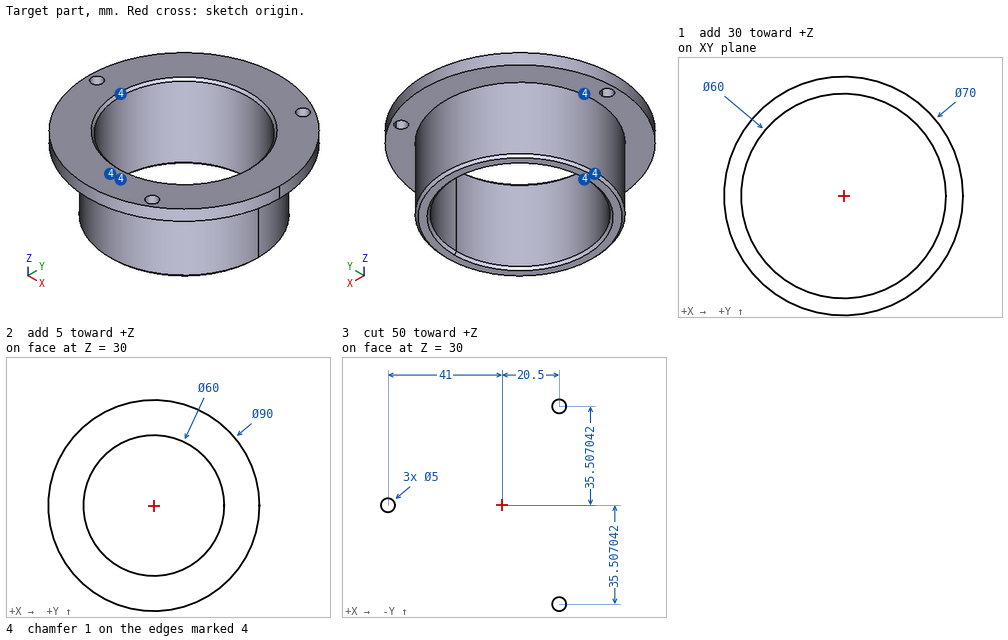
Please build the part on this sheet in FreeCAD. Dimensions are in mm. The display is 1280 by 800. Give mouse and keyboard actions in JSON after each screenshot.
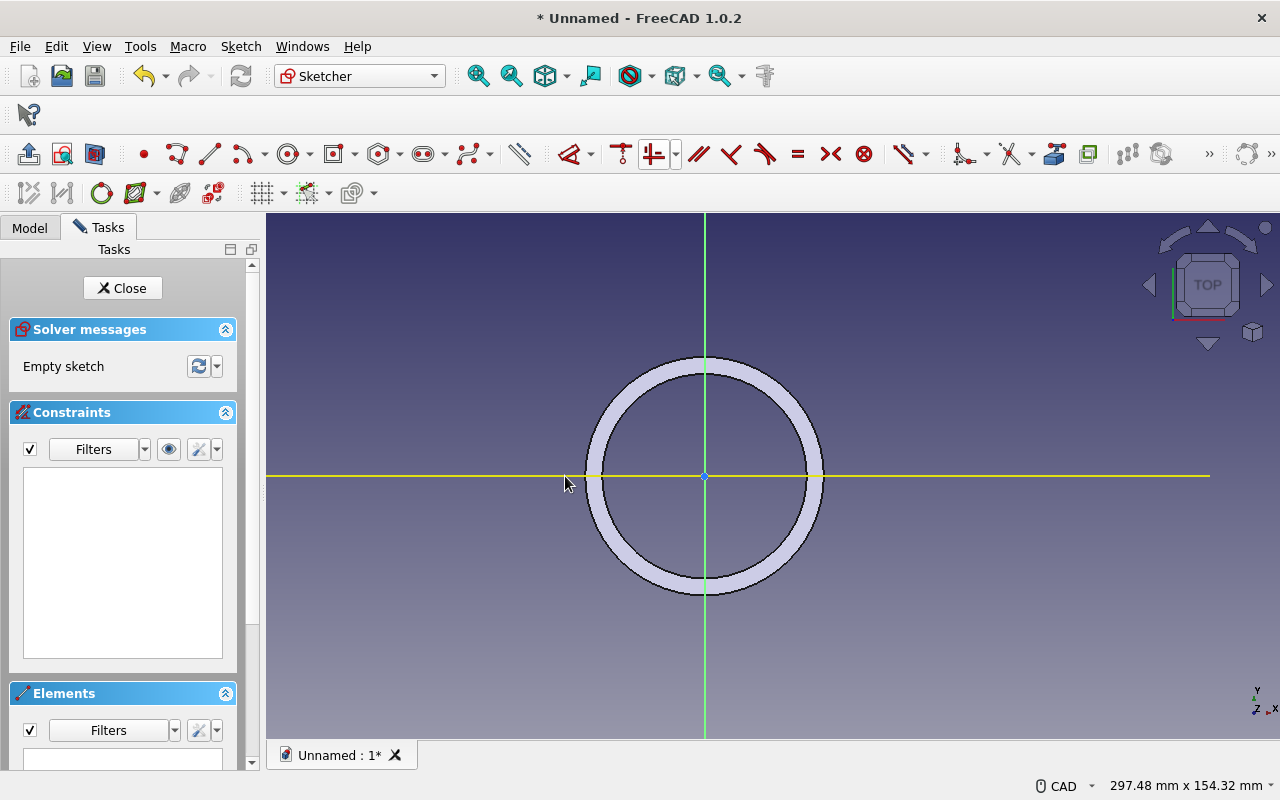
{"action": "left_click", "coordinate": [288, 154]}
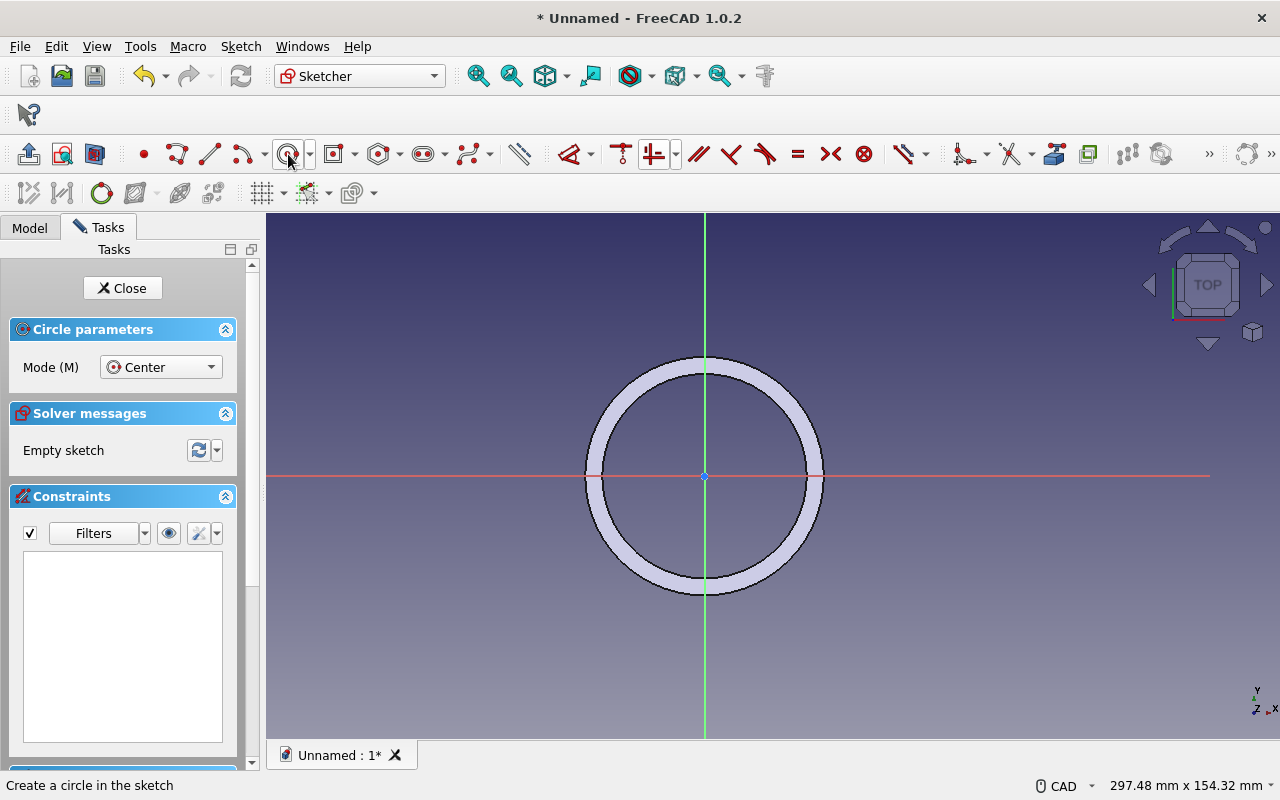
{"action": "left_click", "coordinate": [705, 476]}
{"action": "left_click", "coordinate": [813, 368]}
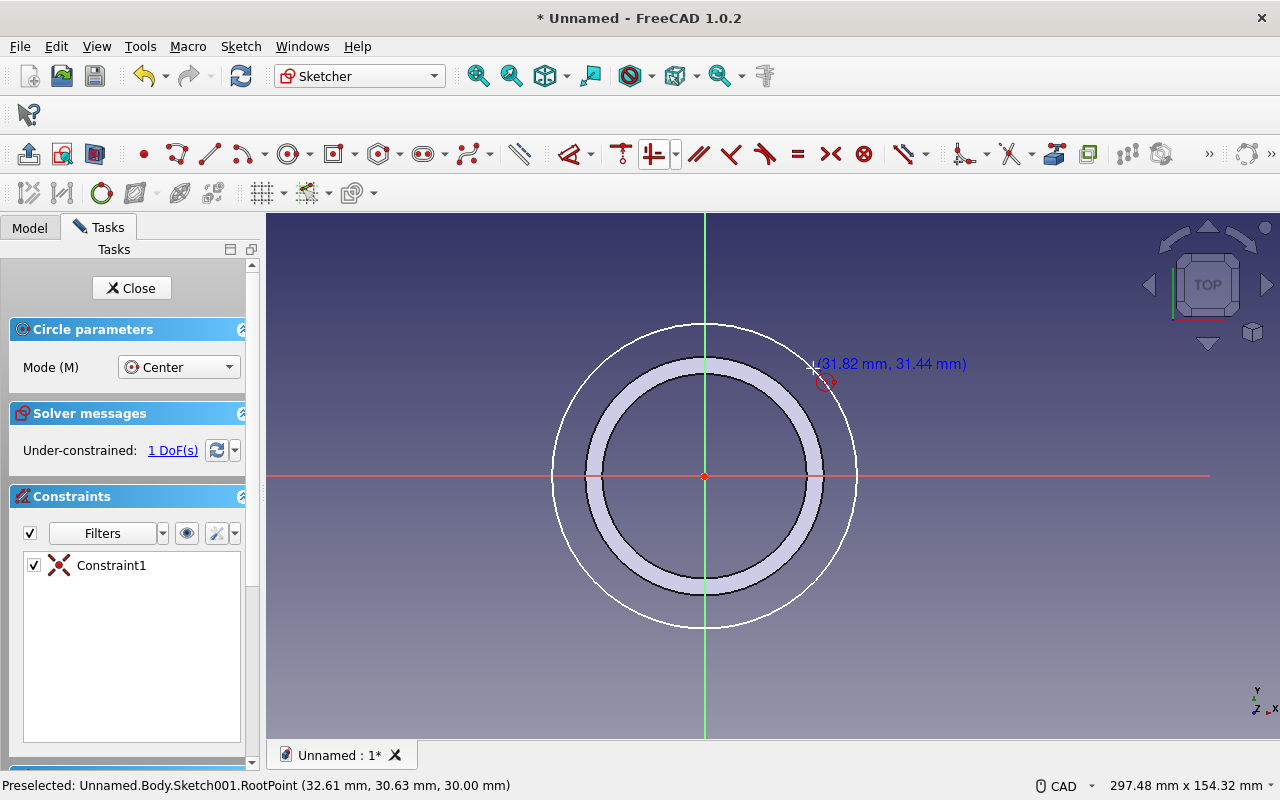
{"action": "left_click", "coordinate": [705, 476]}
{"action": "left_click", "coordinate": [777, 404]}
{"action": "key", "text": "Escape"}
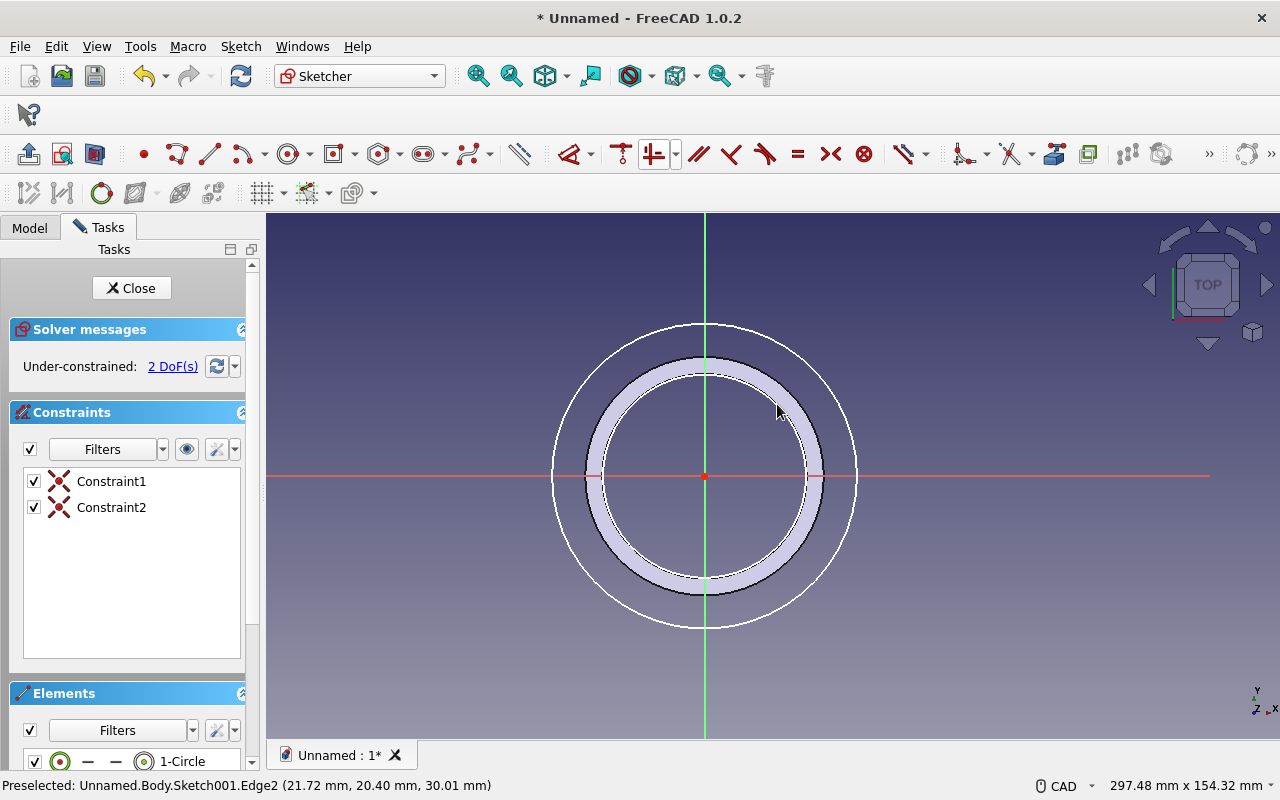
{"action": "left_click", "coordinate": [568, 154]}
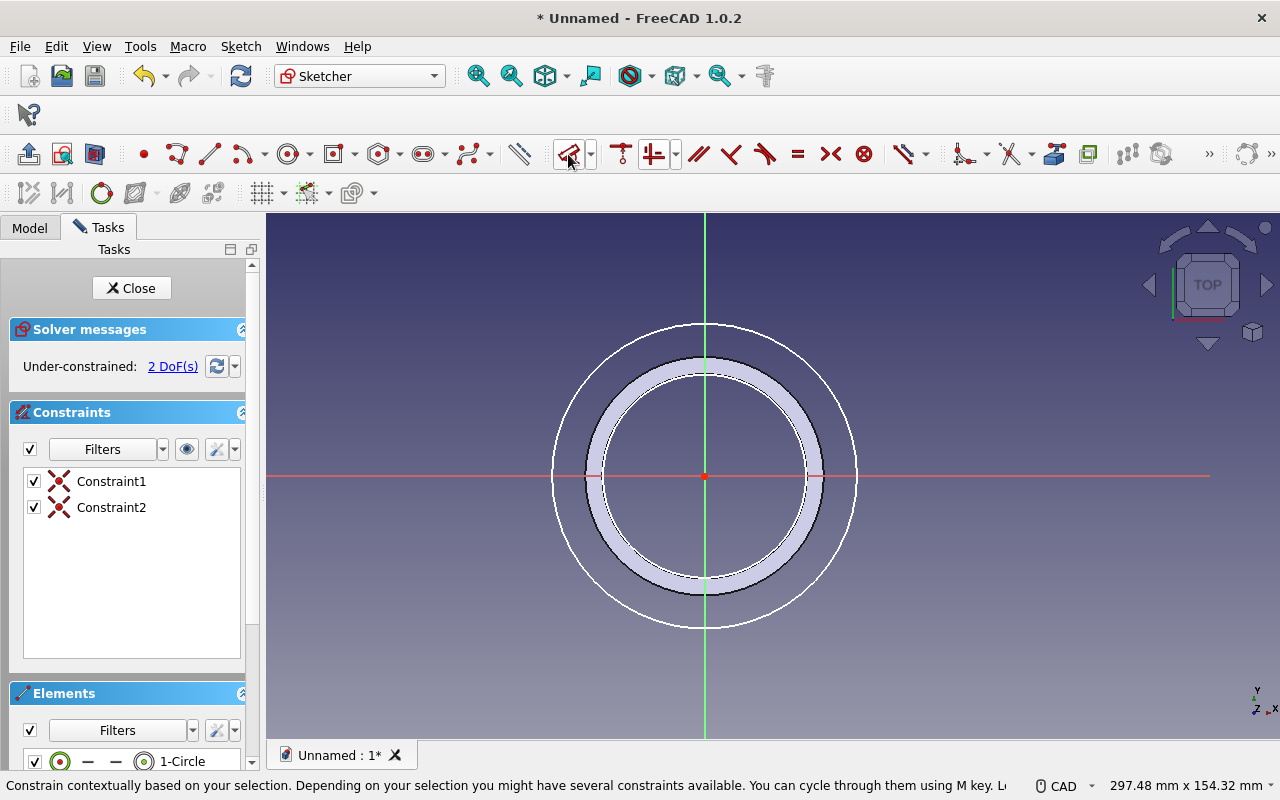
{"action": "left_click", "coordinate": [812, 368]}
{"action": "left_click", "coordinate": [835, 345]}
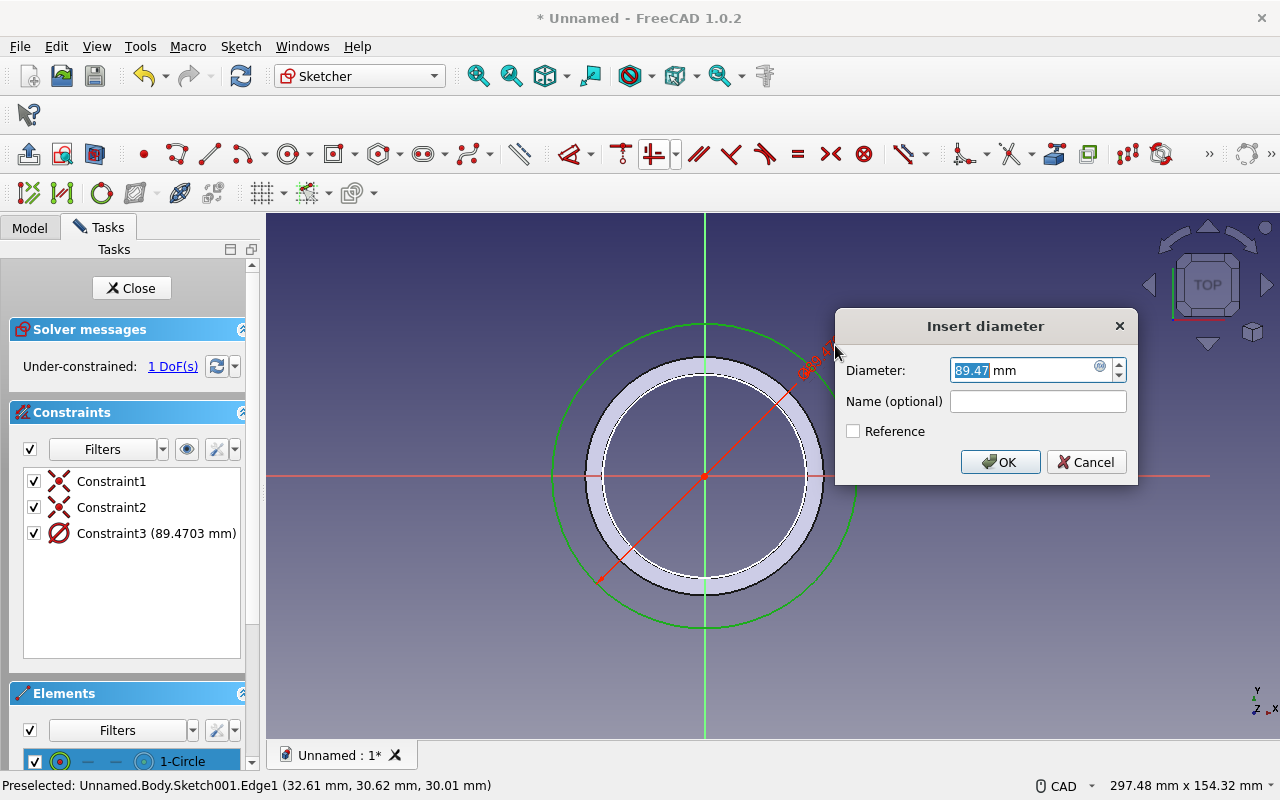
{"action": "type", "text": "90"}
{"action": "key", "text": "Return"}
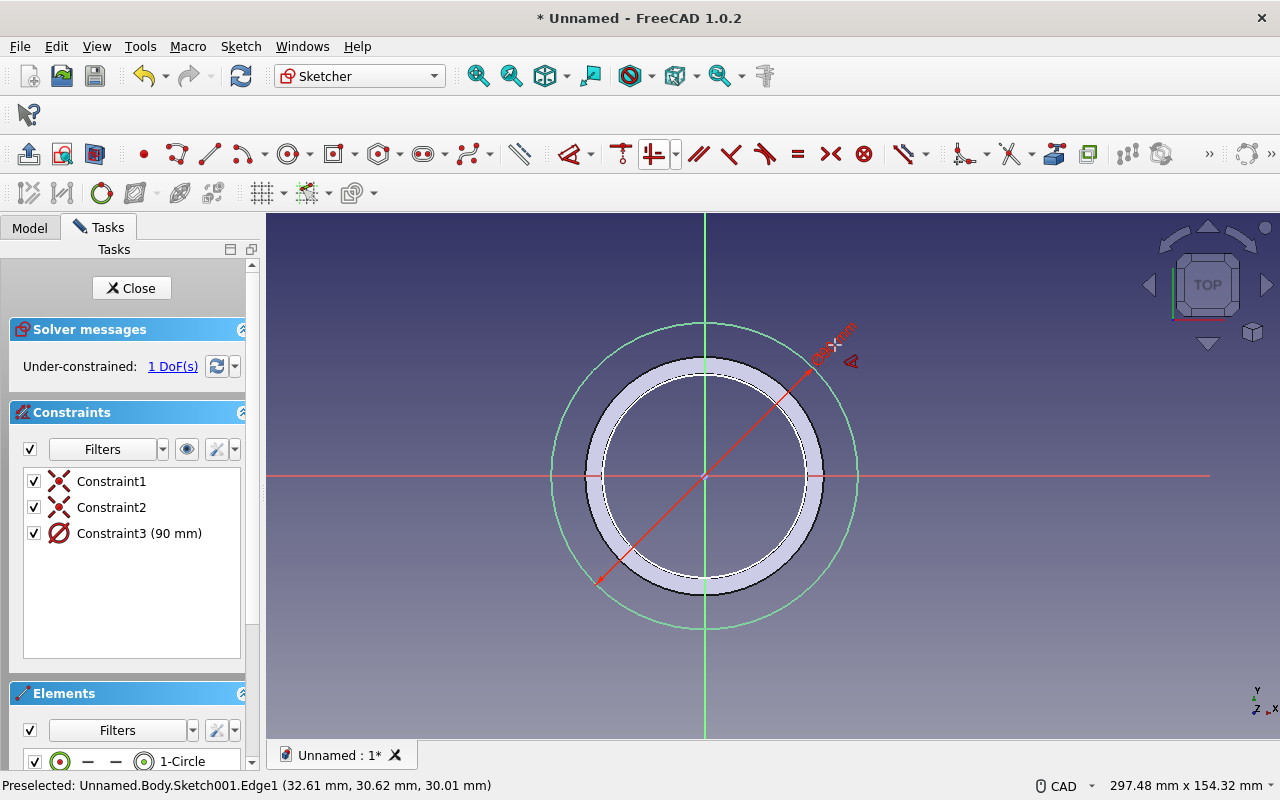
{"action": "left_click", "coordinate": [776, 404]}
{"action": "left_click", "coordinate": [799, 381]}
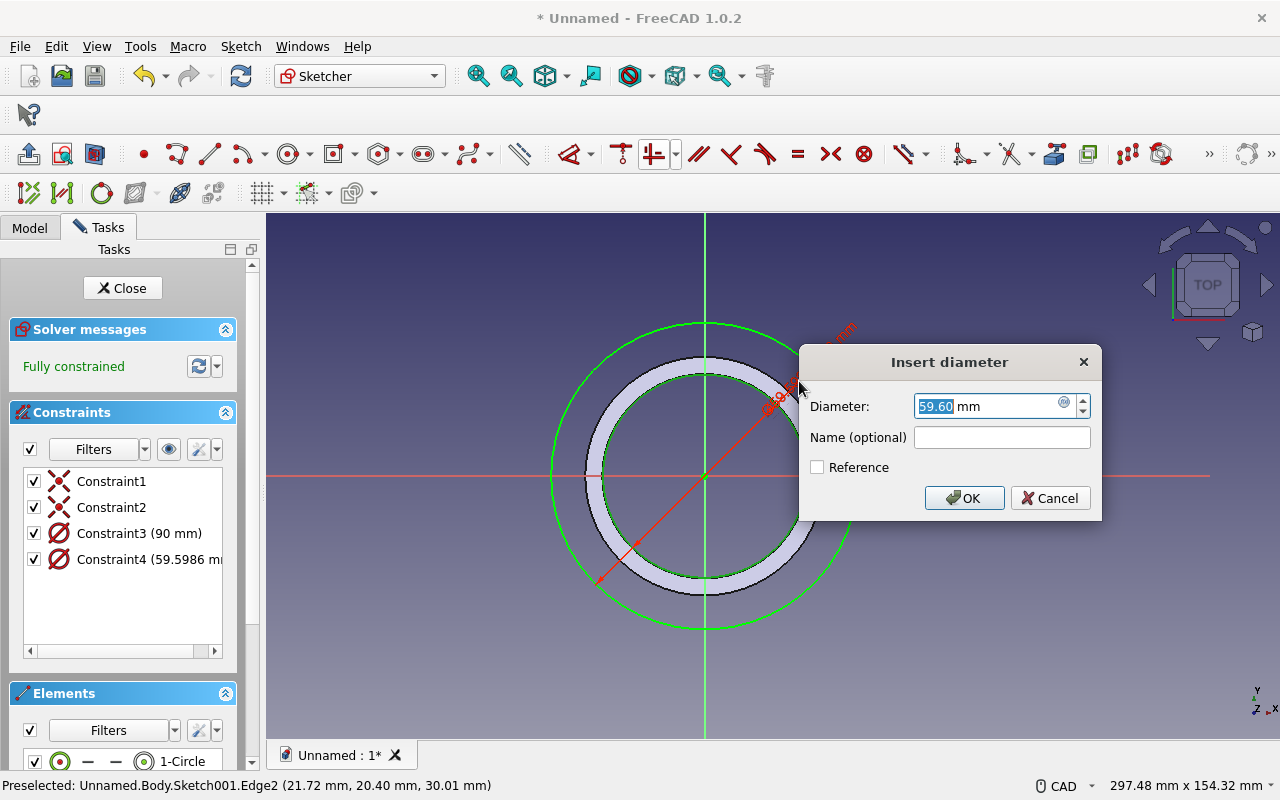
{"action": "type", "text": "60"}
{"action": "key", "text": "Return"}
{"action": "key", "text": "Escape"}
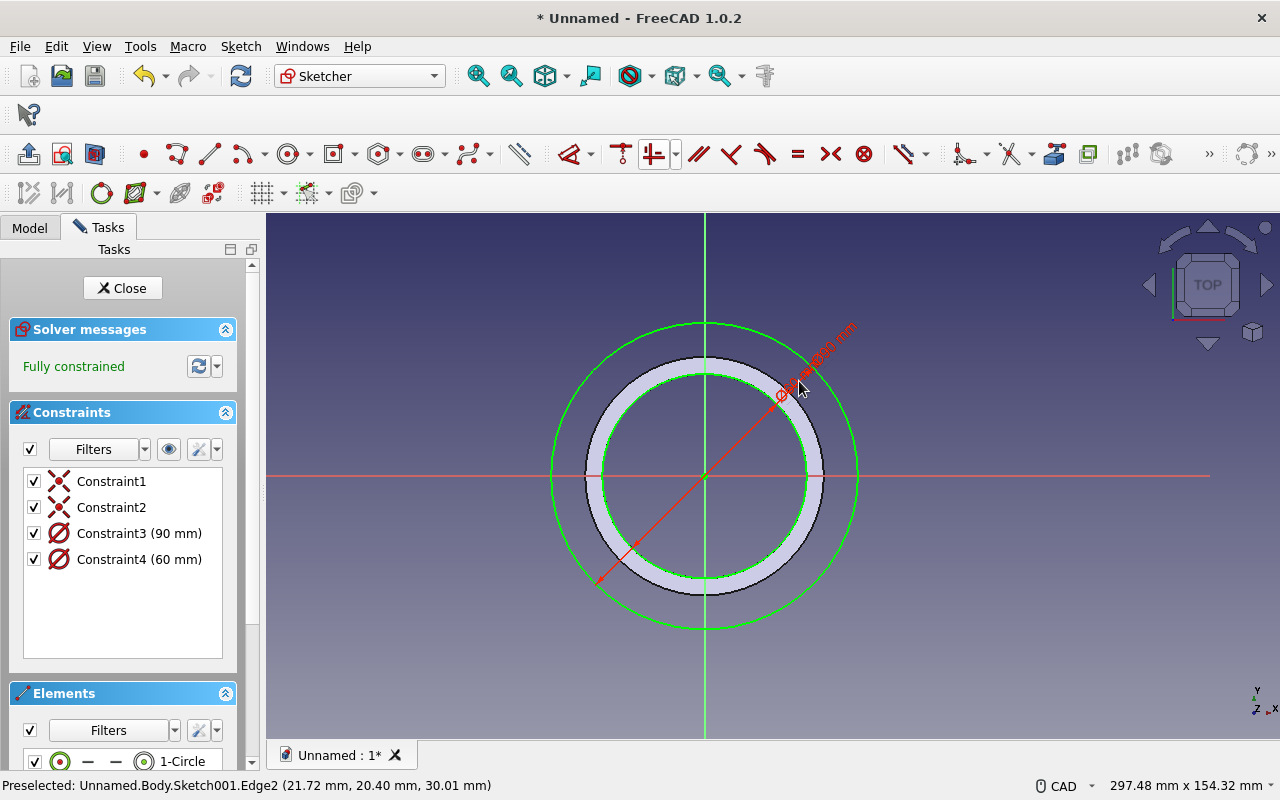
{"action": "left_click", "coordinate": [123, 288]}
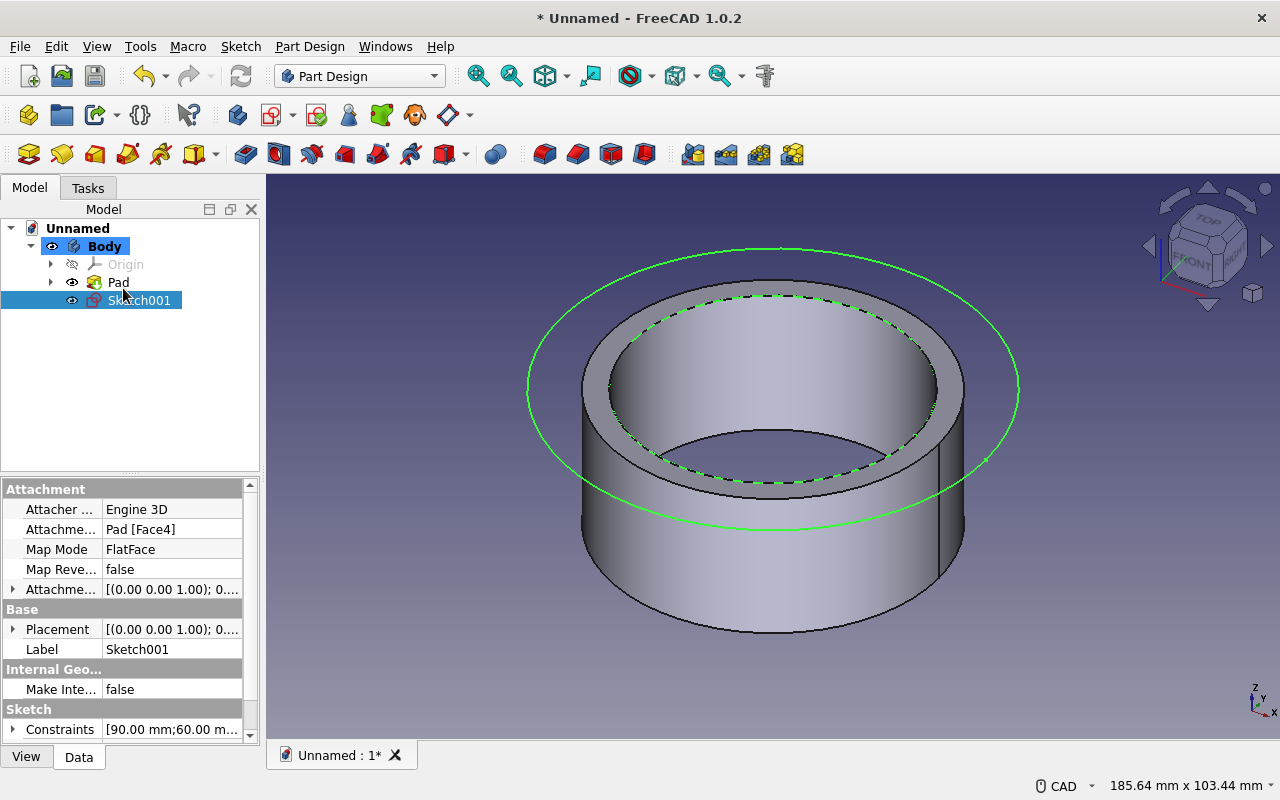
{"action": "left_click", "coordinate": [29, 154]}